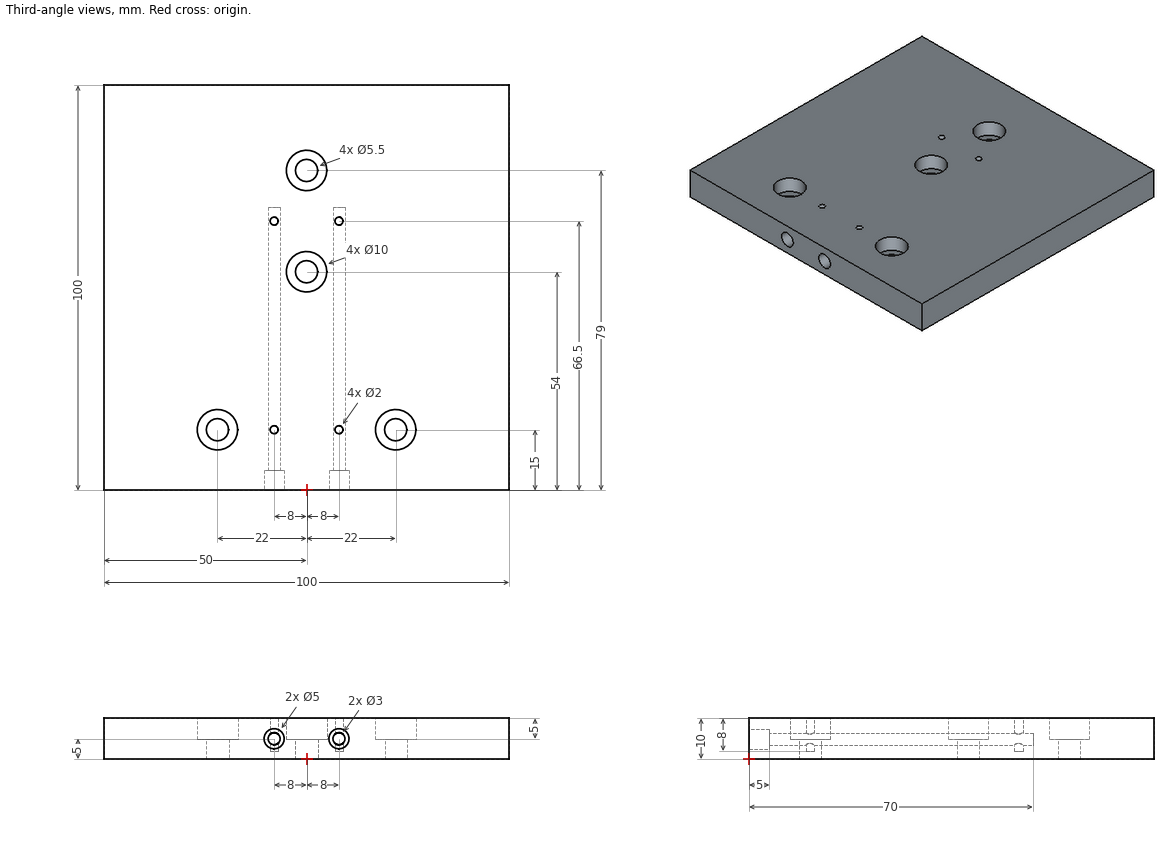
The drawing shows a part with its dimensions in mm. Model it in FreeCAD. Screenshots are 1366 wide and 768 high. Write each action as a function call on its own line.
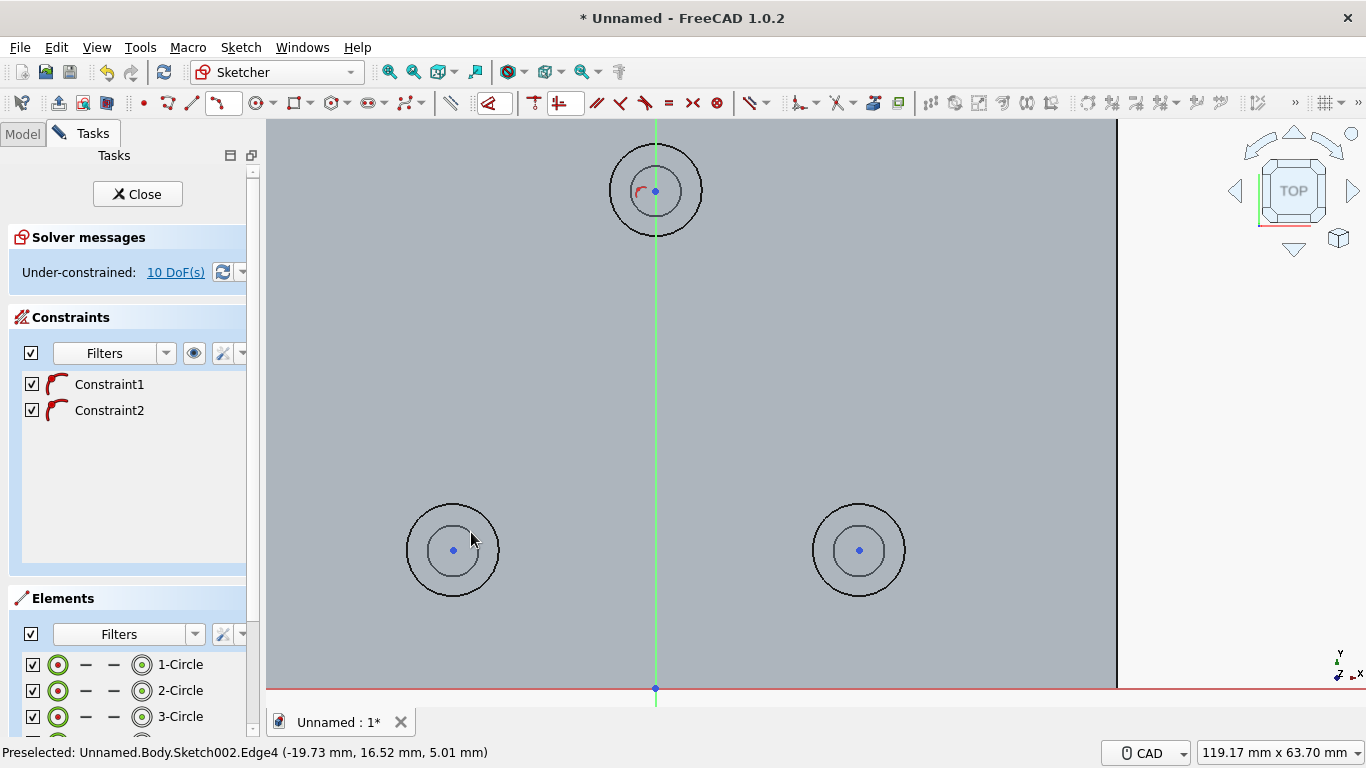
scroll(859, 537, down, 3)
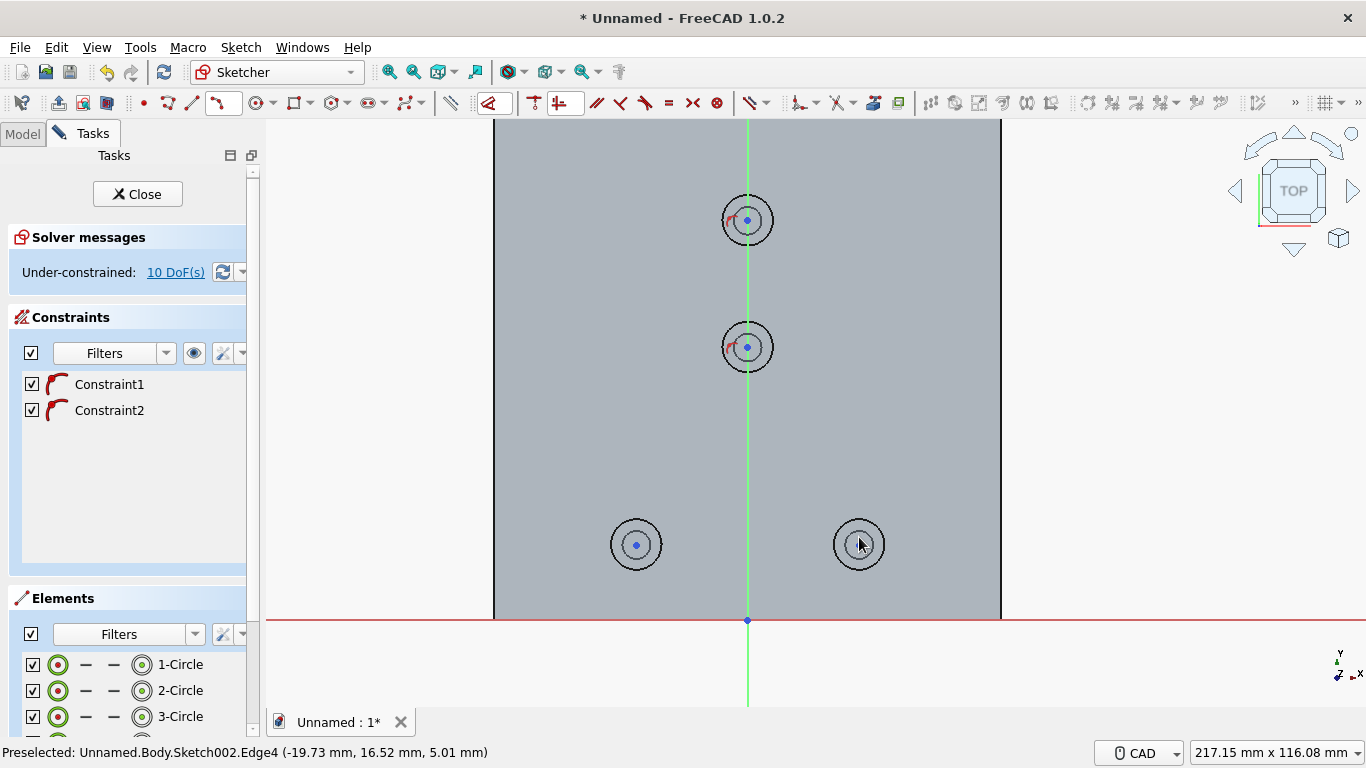
scroll(757, 211, up, 2)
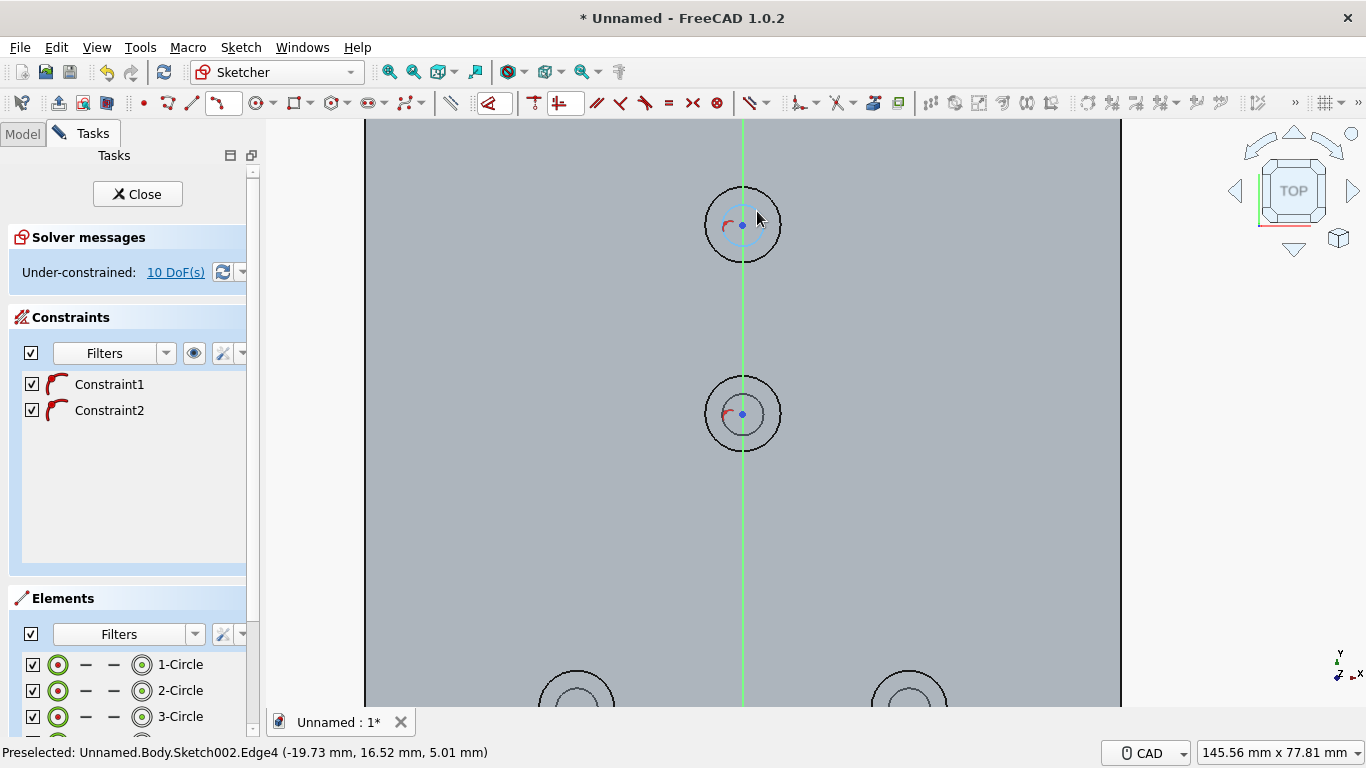
click(757, 211)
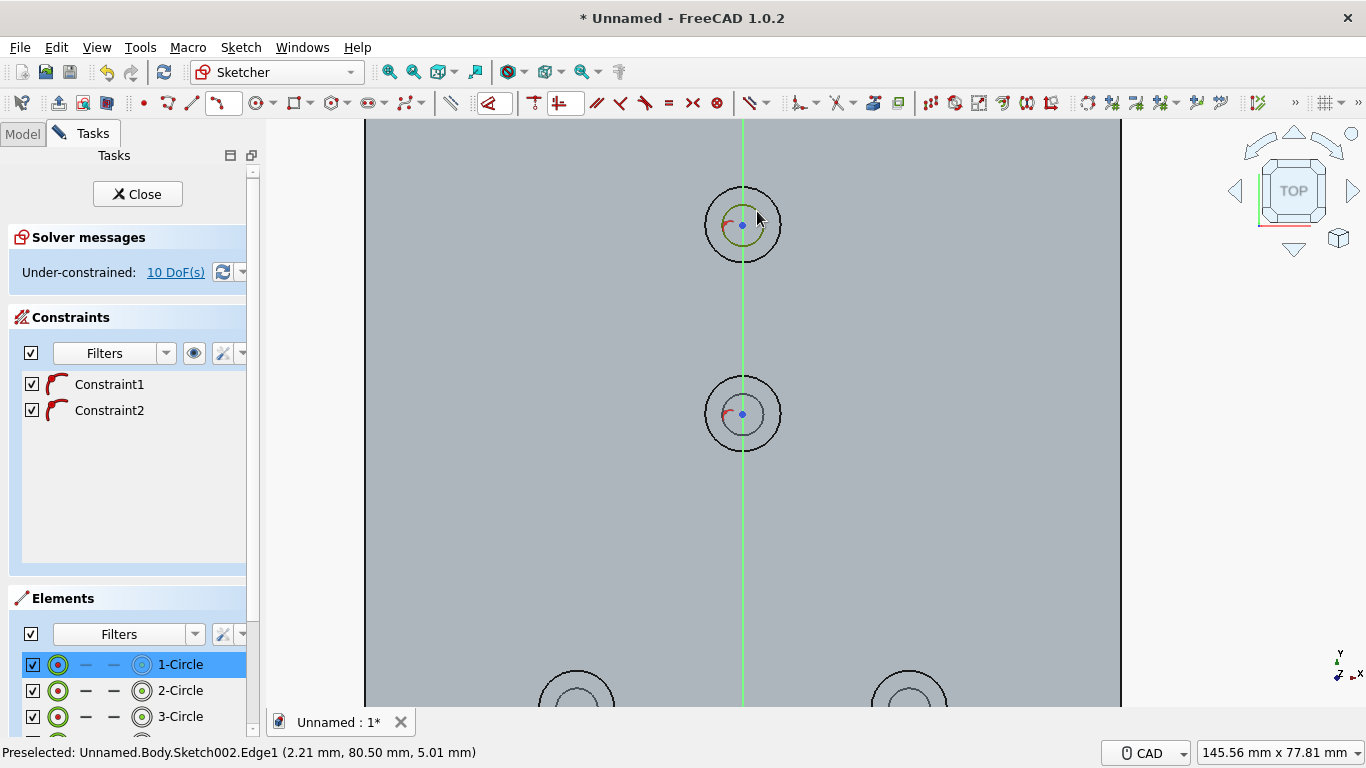
click(757, 400)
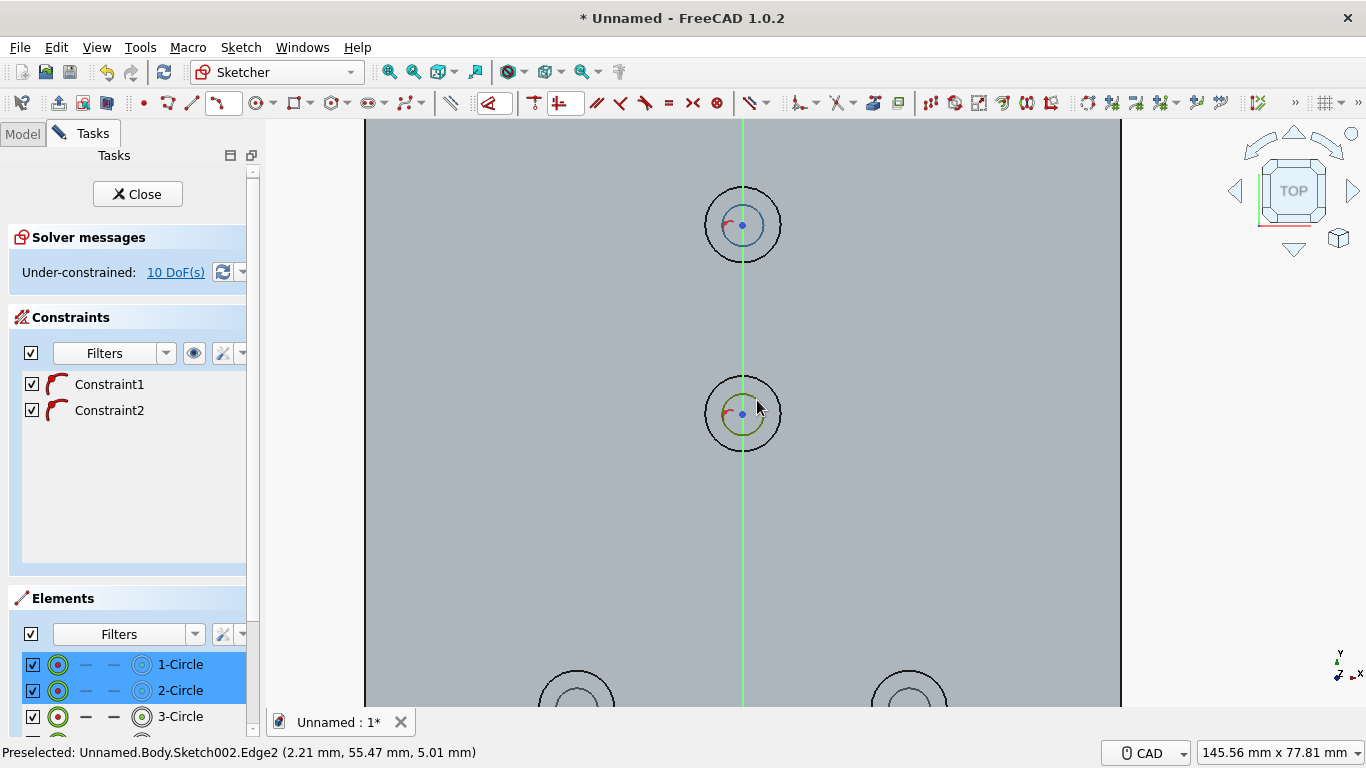
scroll(757, 210, down, 2)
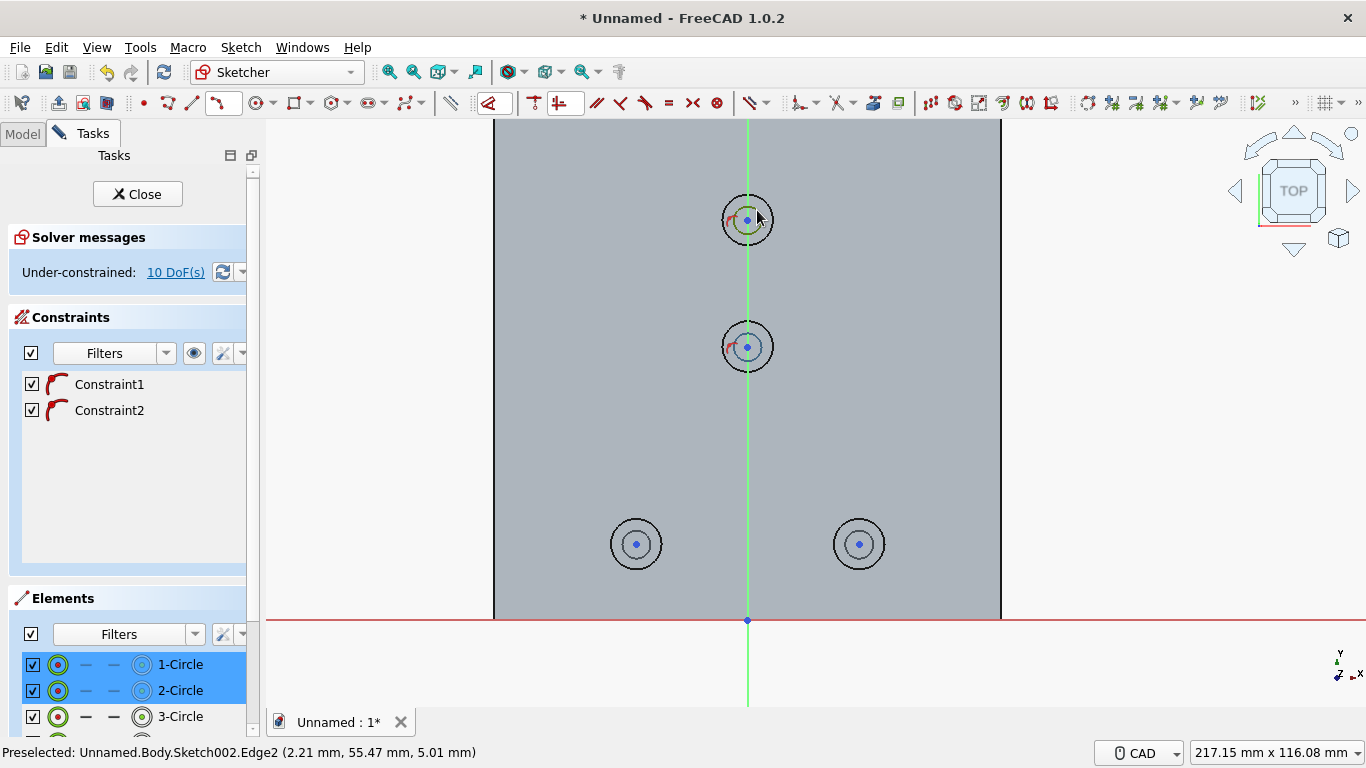
click(869, 535)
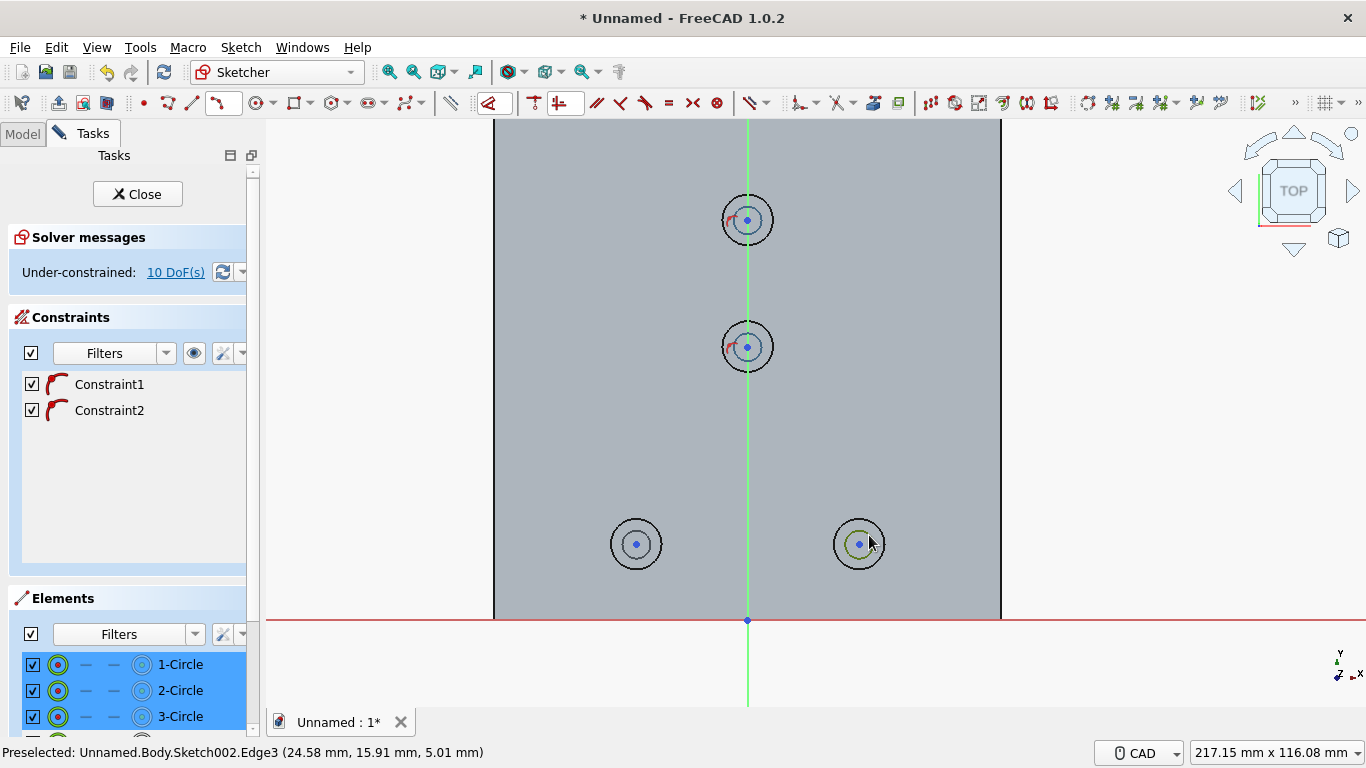
click(646, 535)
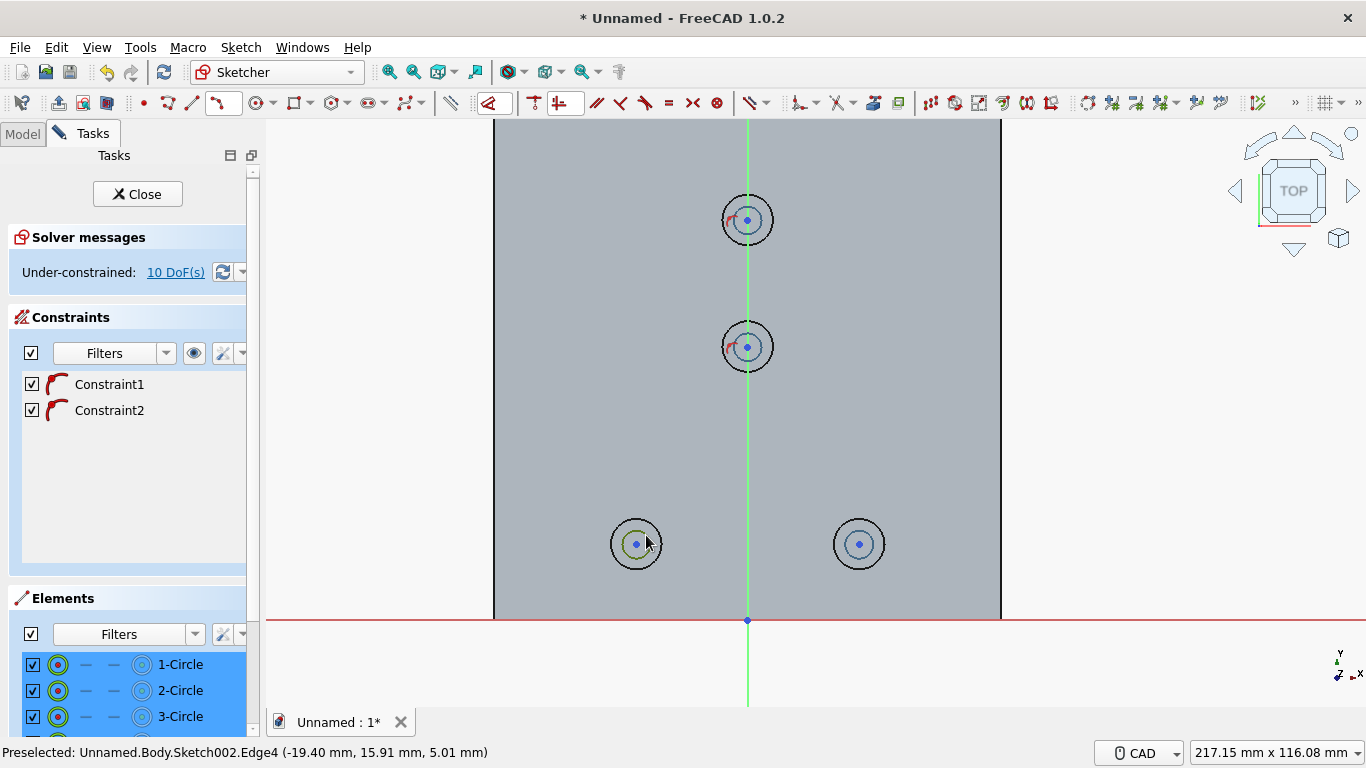
click(670, 104)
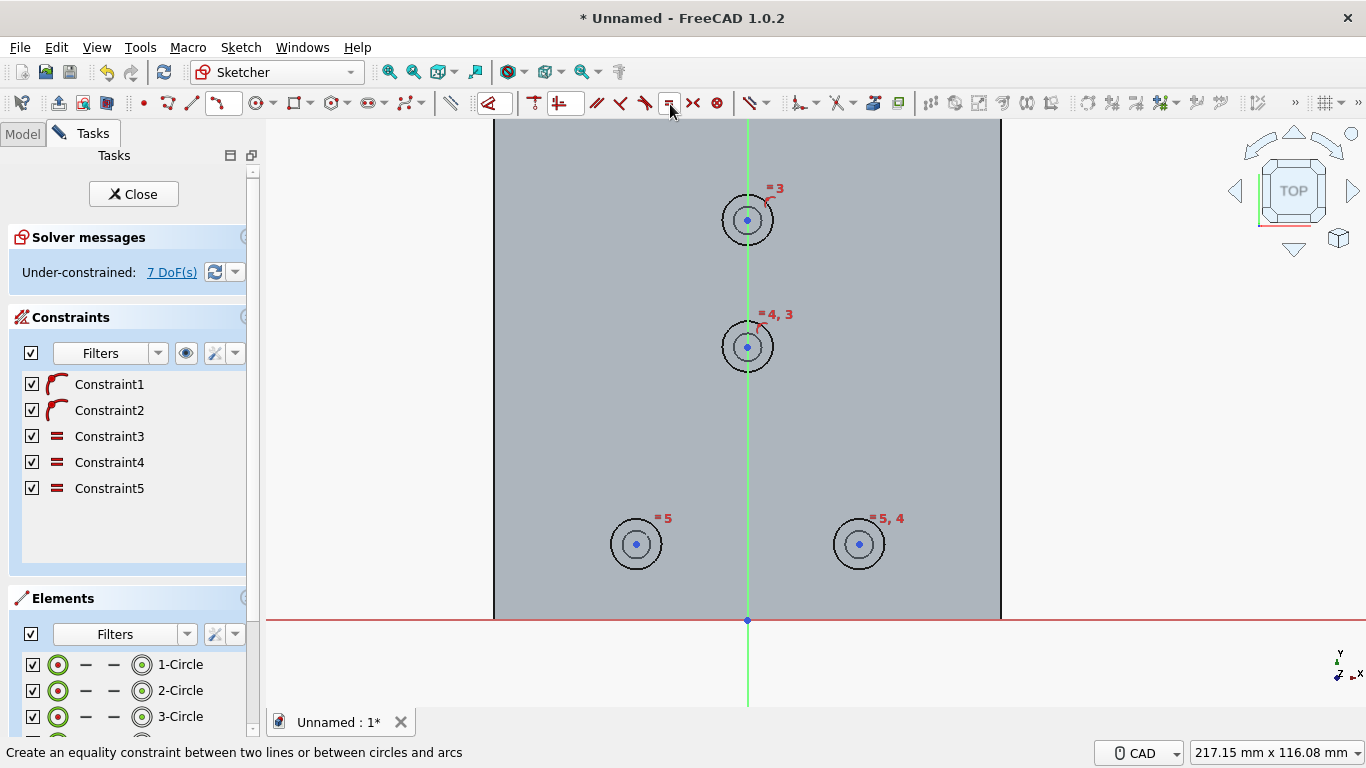
scroll(757, 211, up, 2)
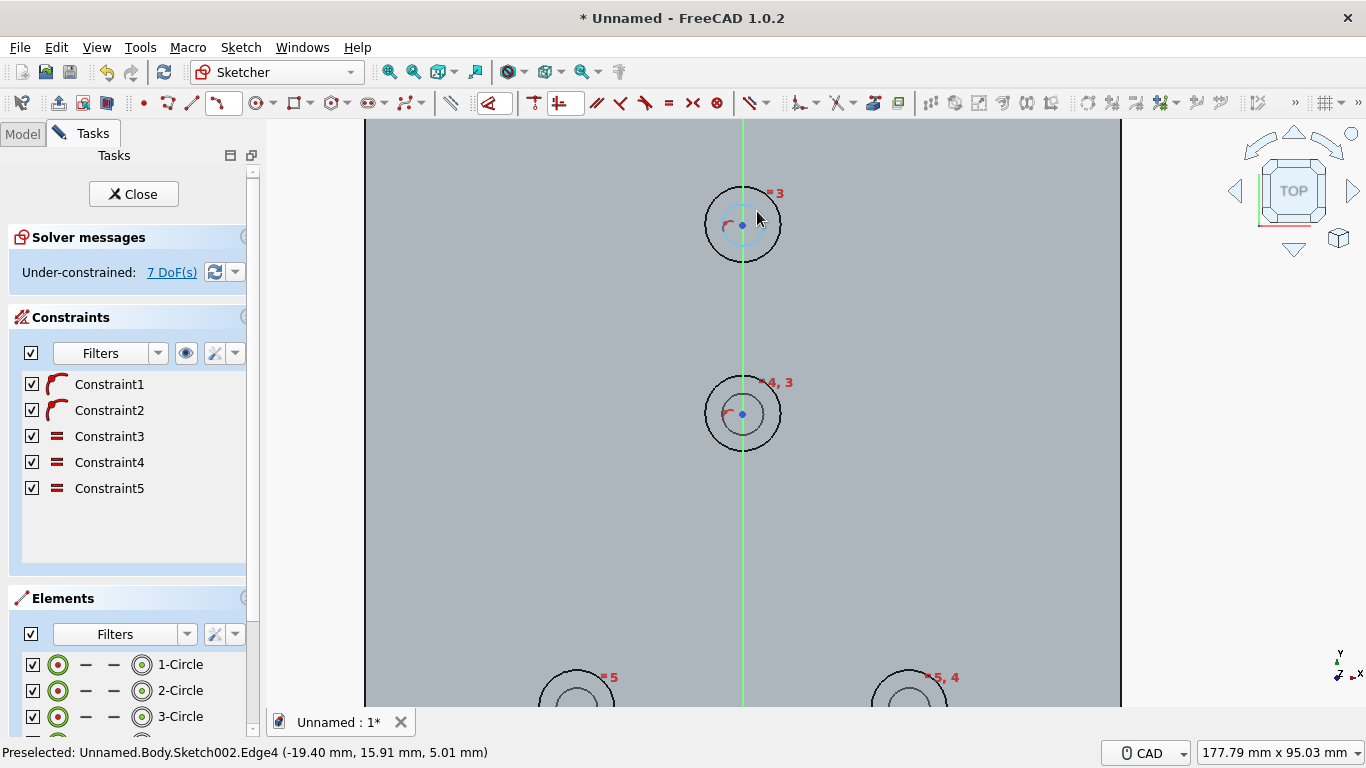
click(757, 210)